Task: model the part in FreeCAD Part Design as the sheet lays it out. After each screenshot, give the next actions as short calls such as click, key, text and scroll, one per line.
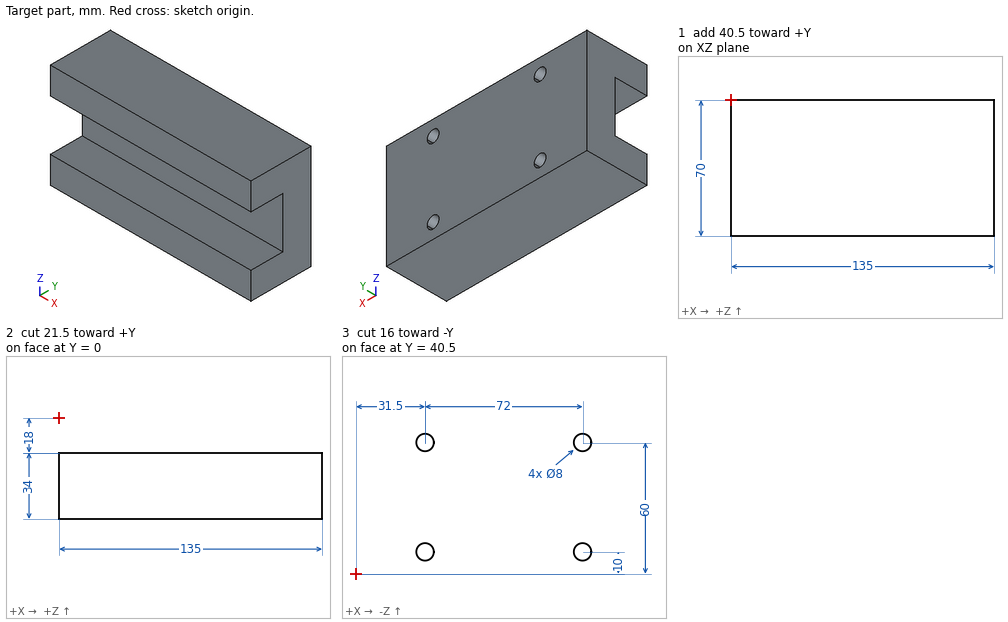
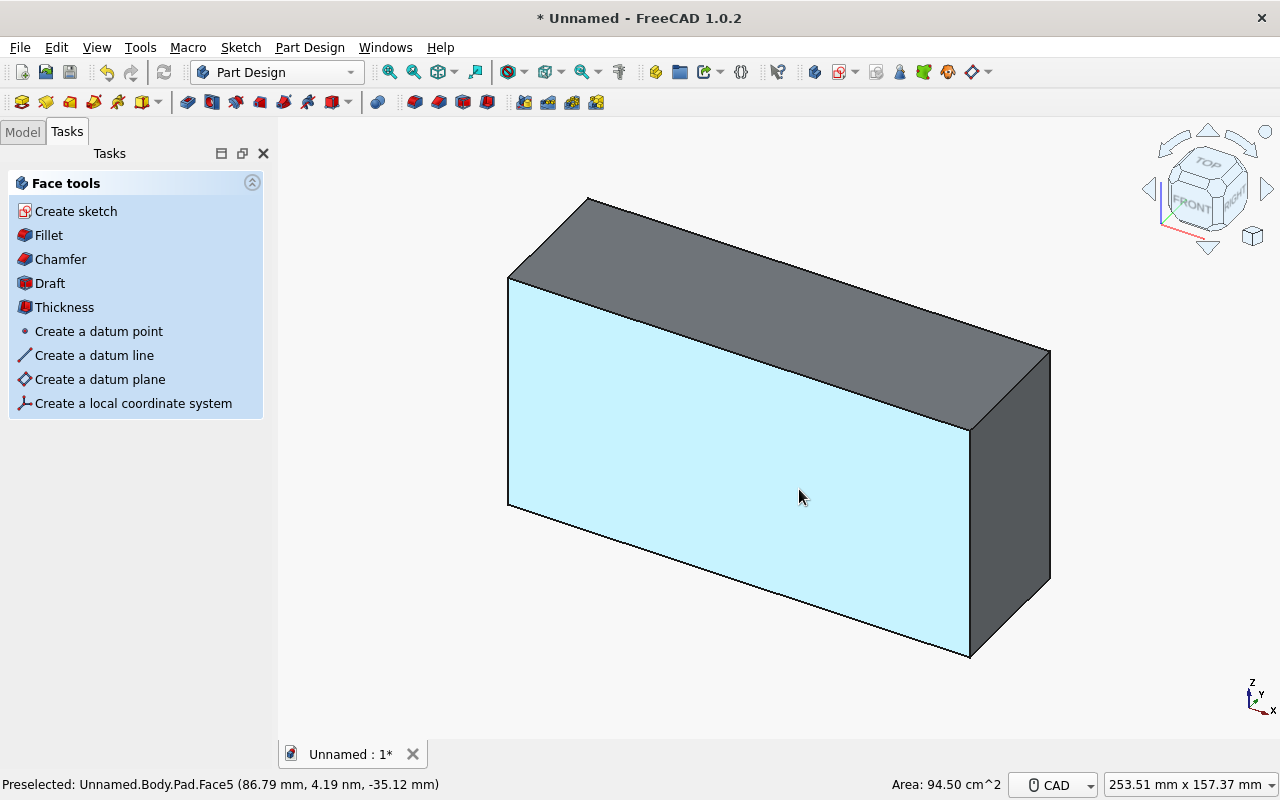
click(840, 72)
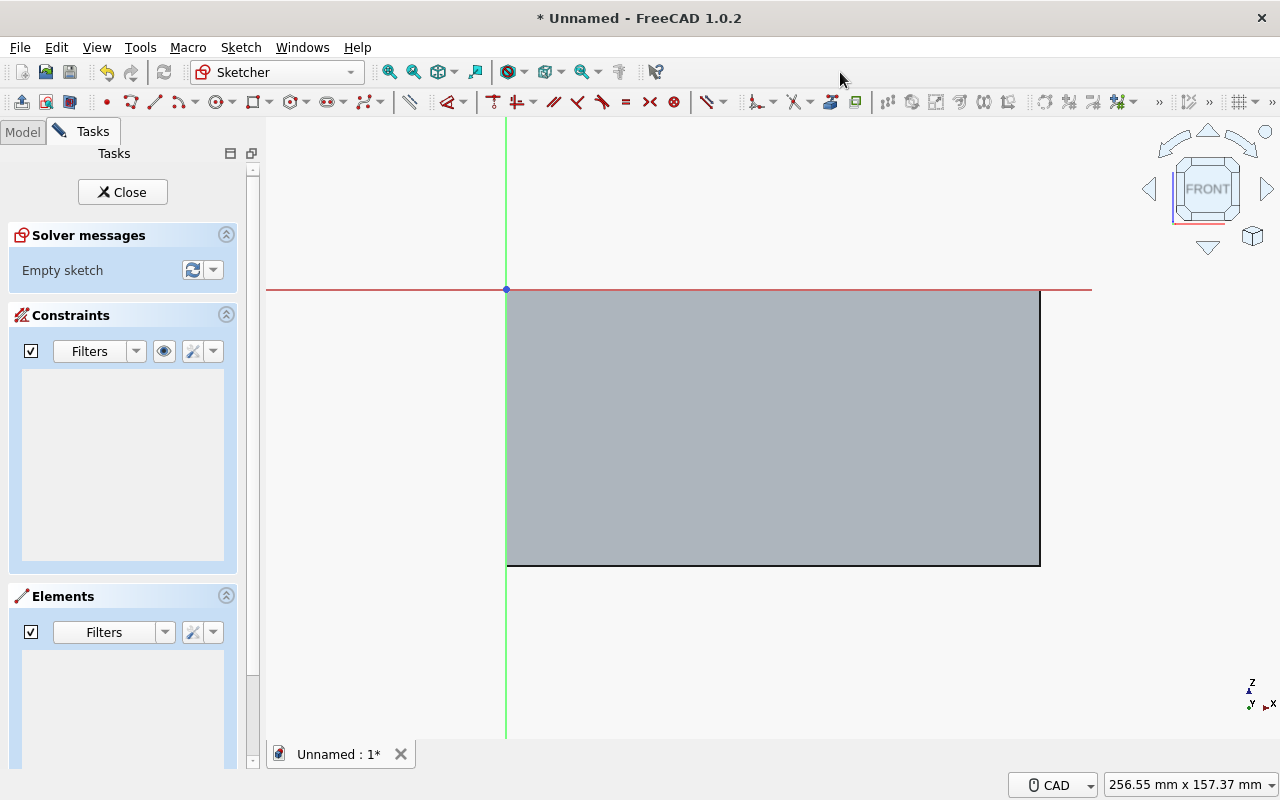
click(254, 102)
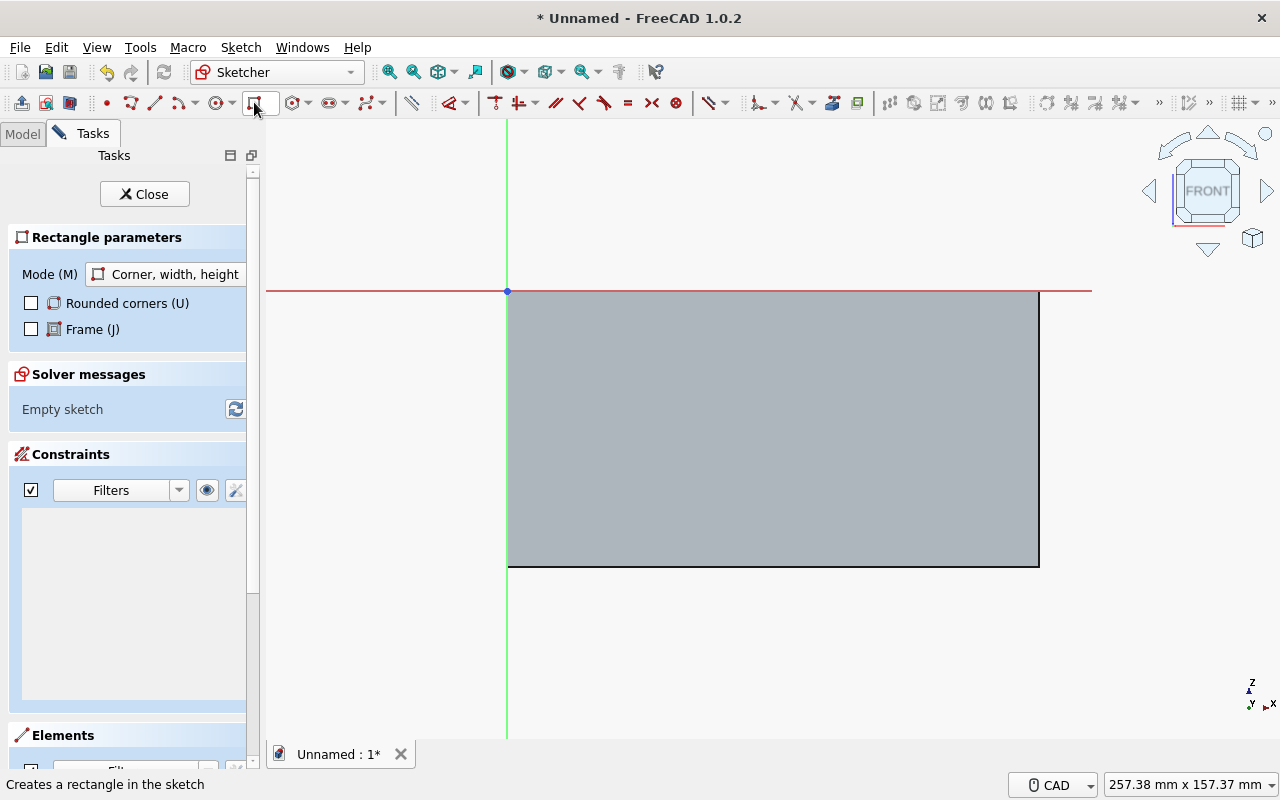
click(507, 362)
click(1039, 496)
key(Escape)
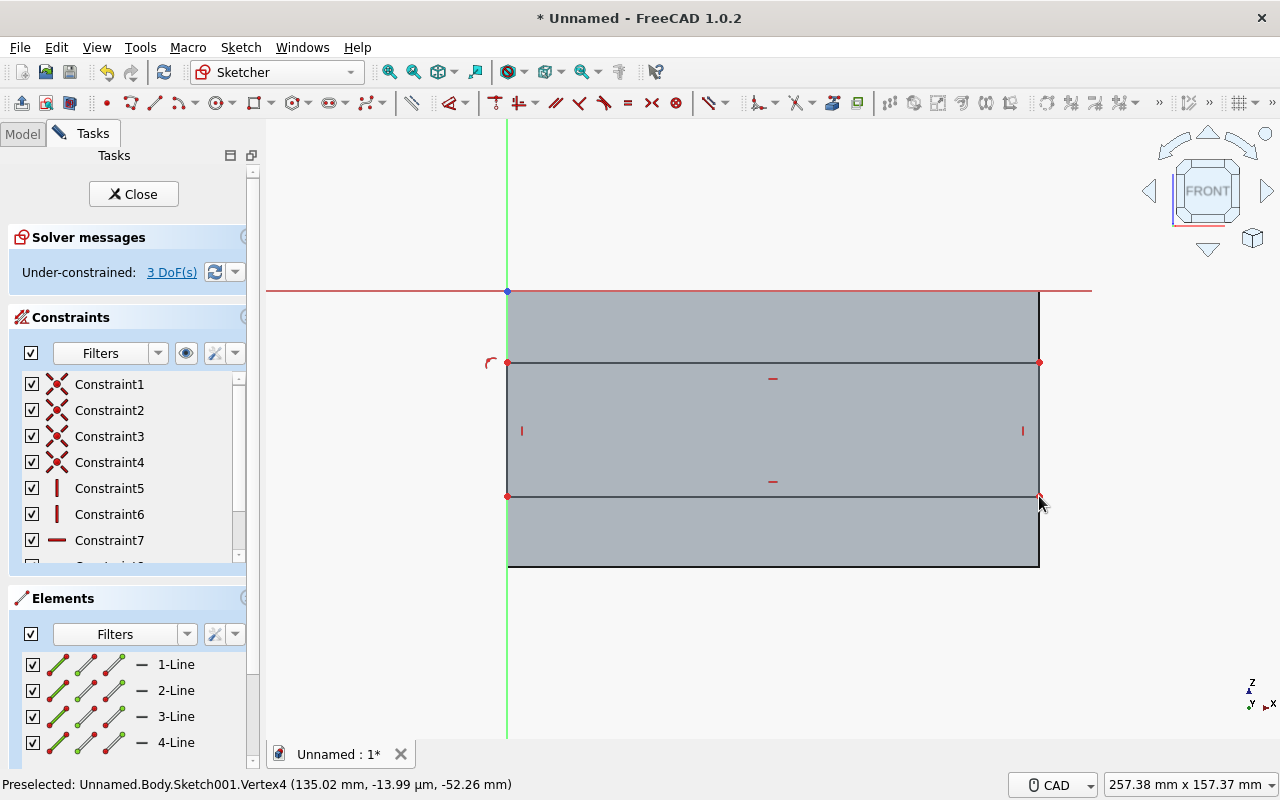
click(507, 403)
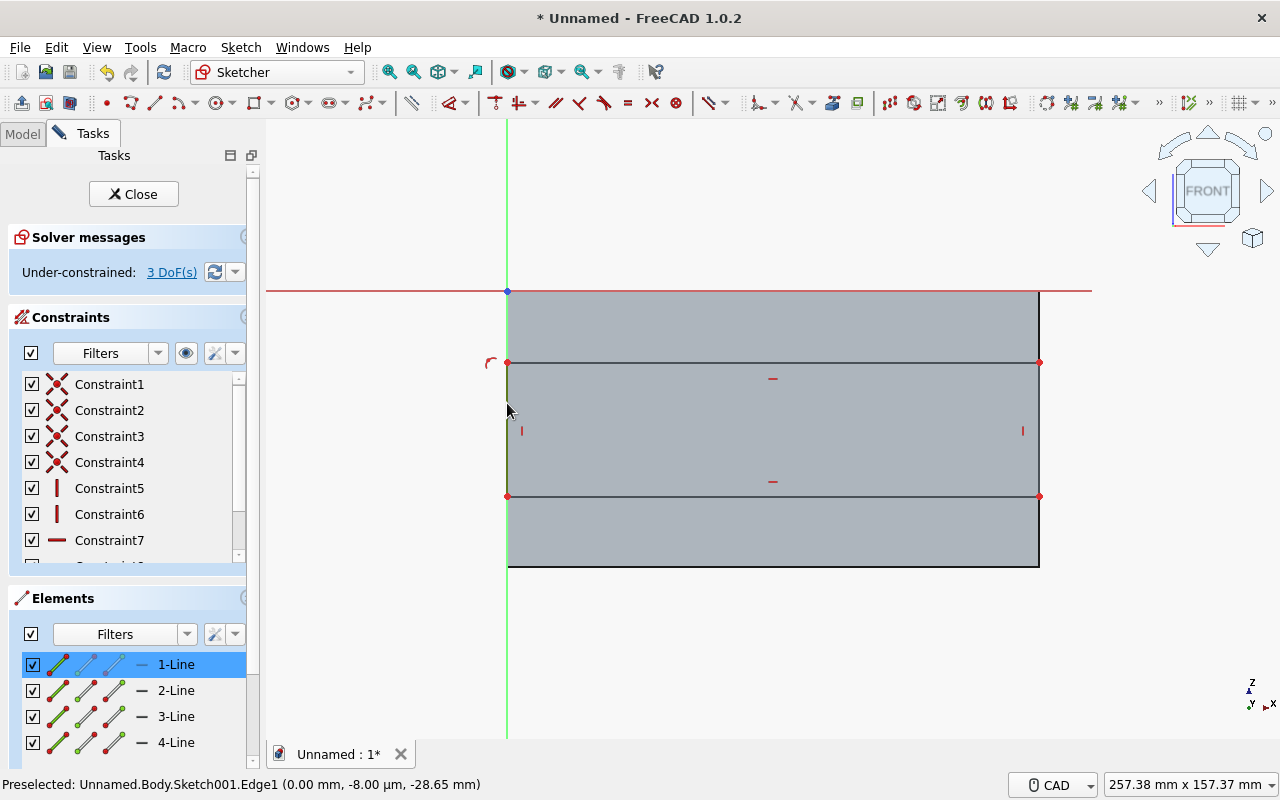
click(468, 104)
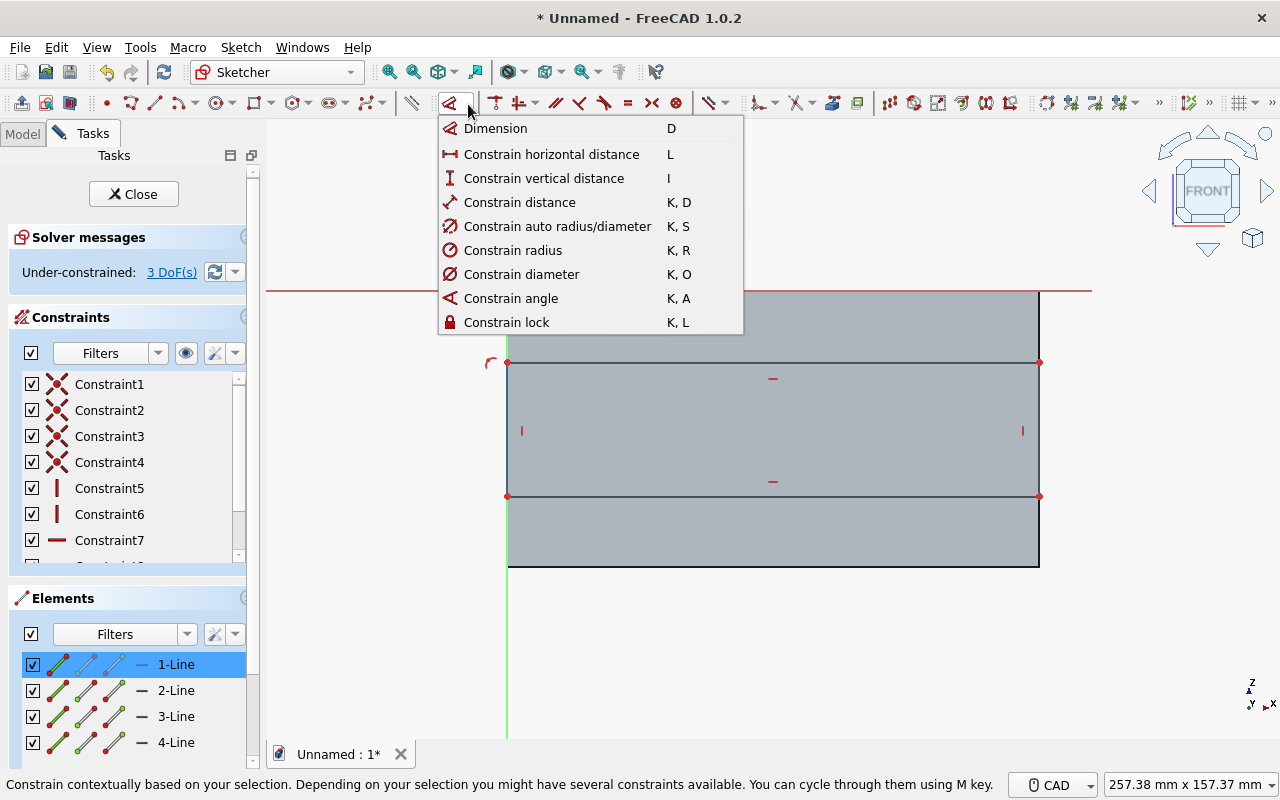
click(591, 178)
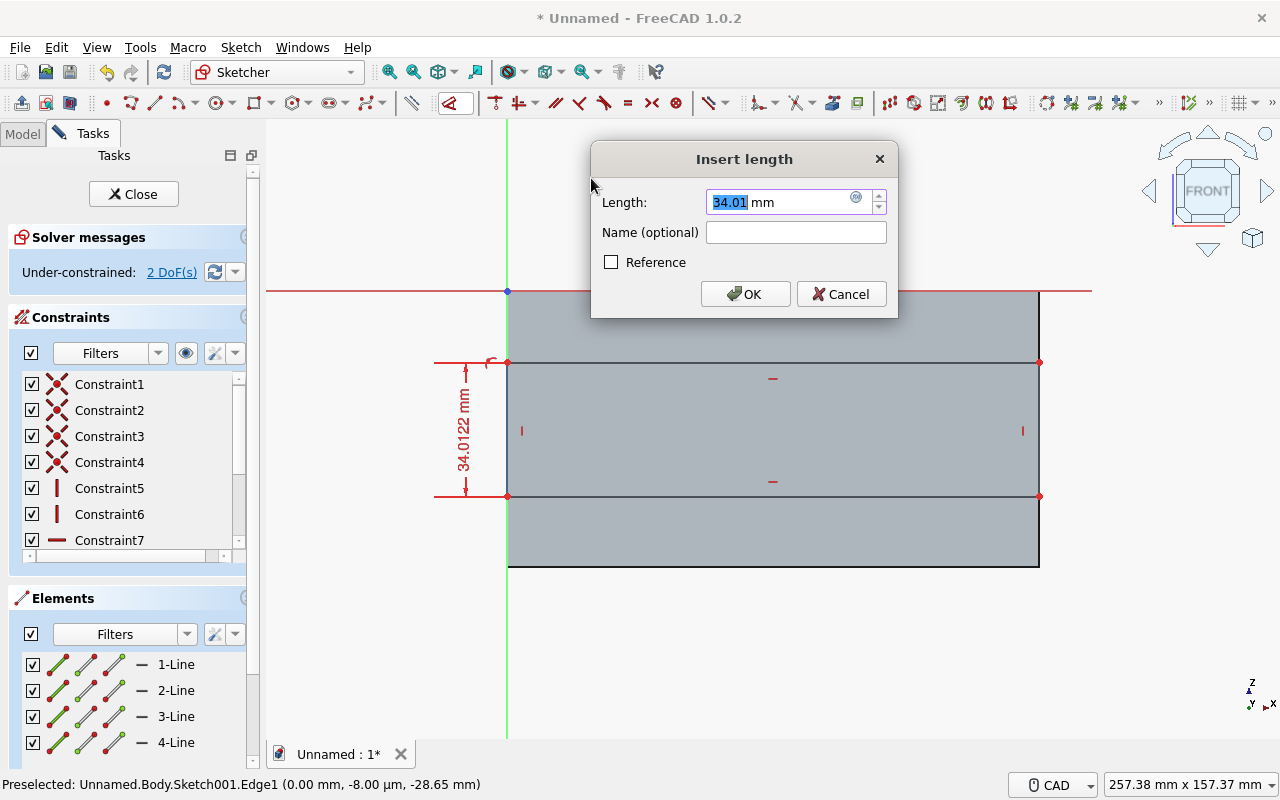
text(34)
key(Return)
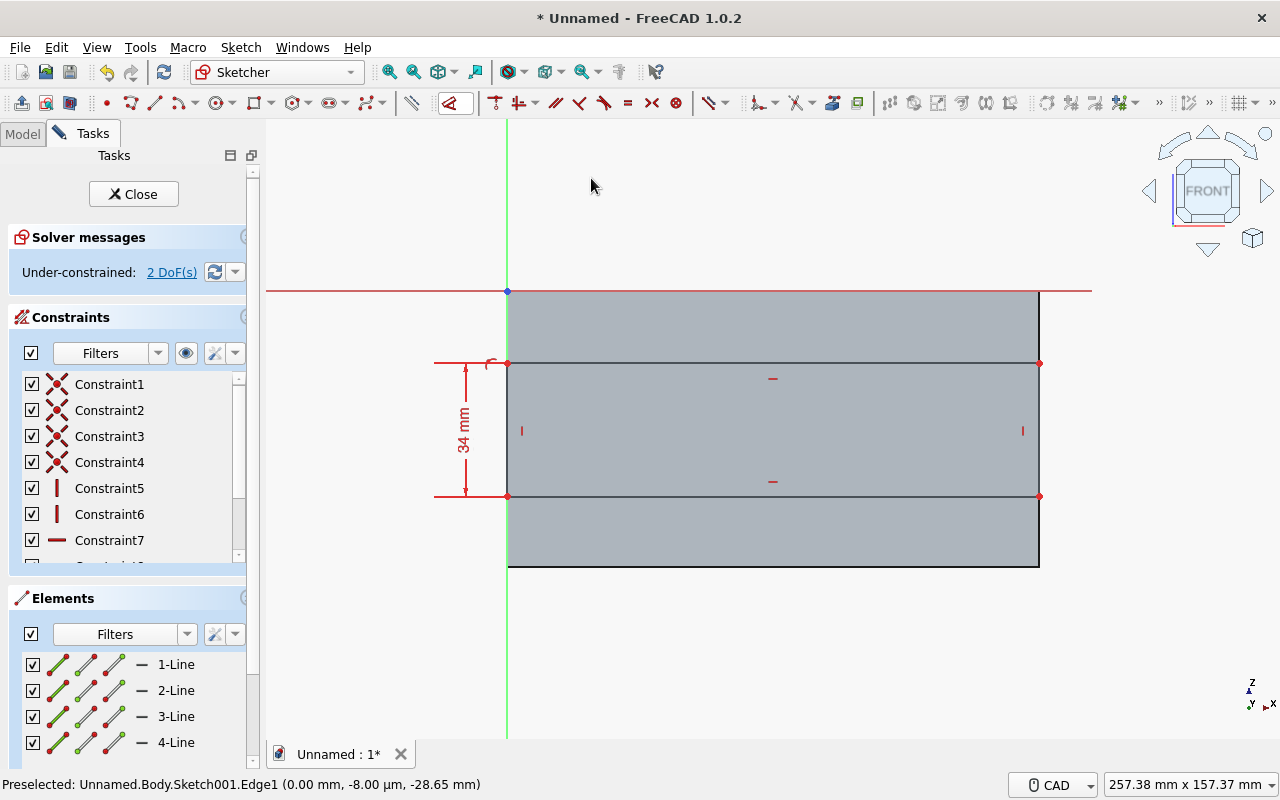
click(667, 497)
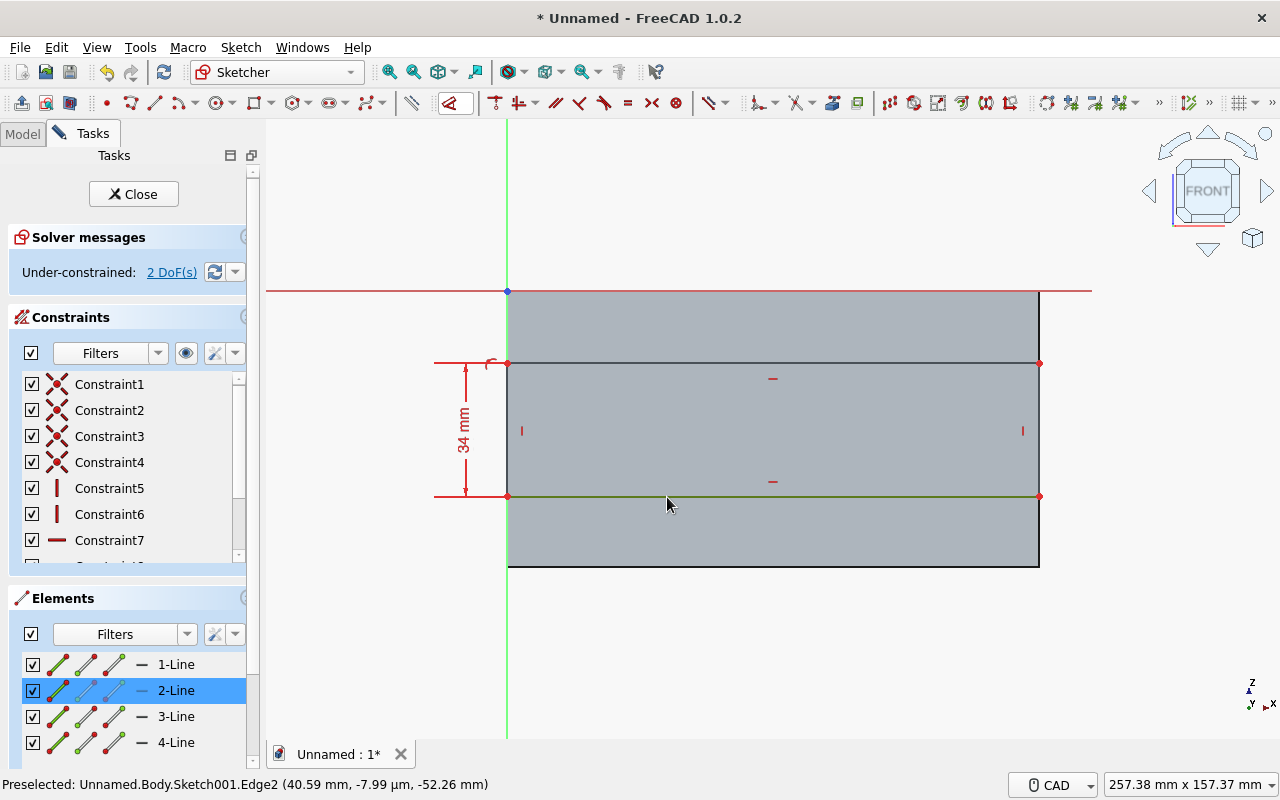
key(l)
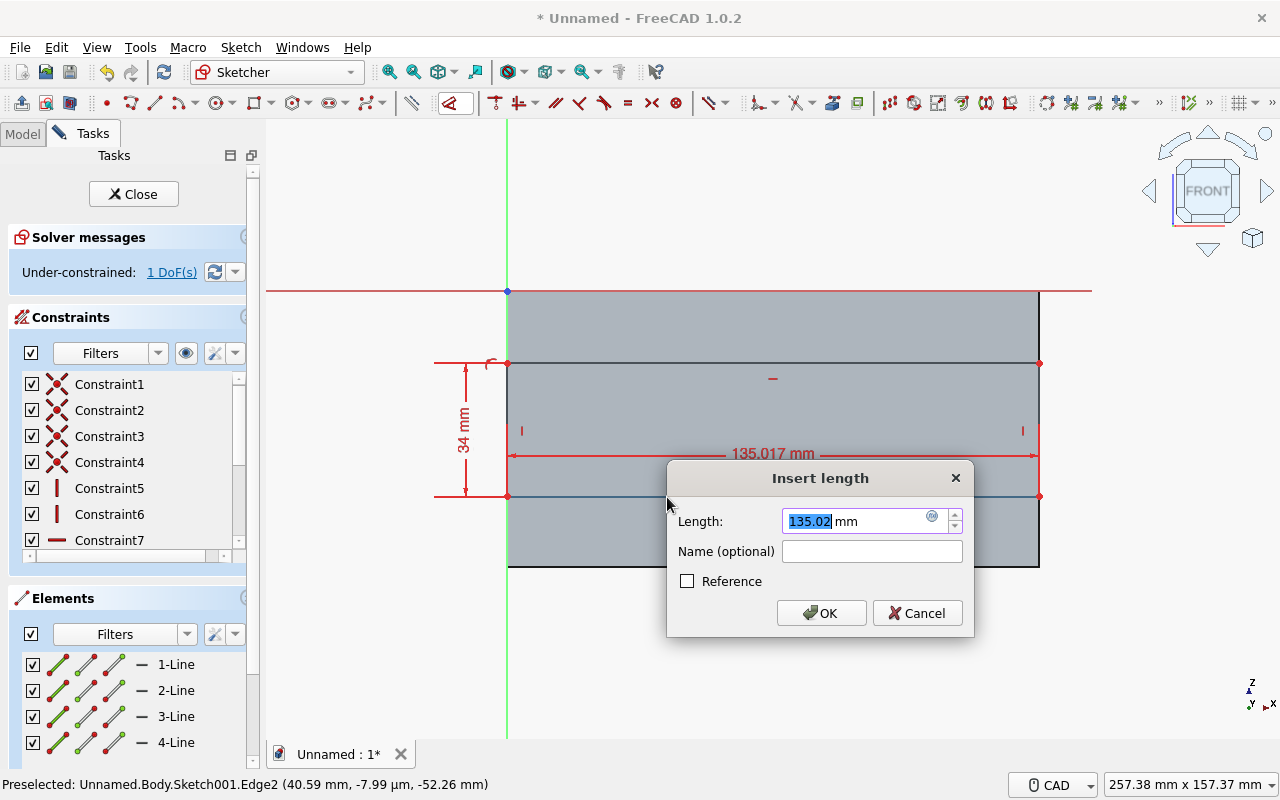
text(135)
key(Return)